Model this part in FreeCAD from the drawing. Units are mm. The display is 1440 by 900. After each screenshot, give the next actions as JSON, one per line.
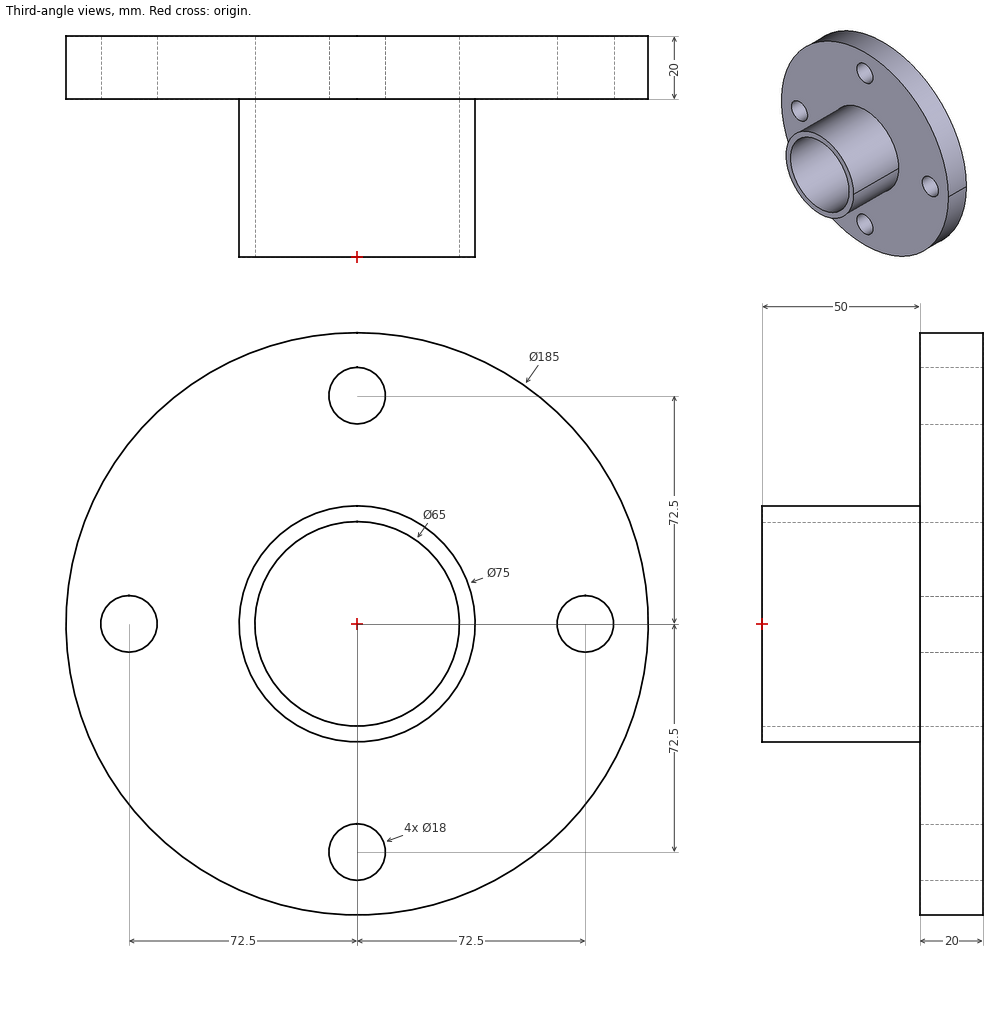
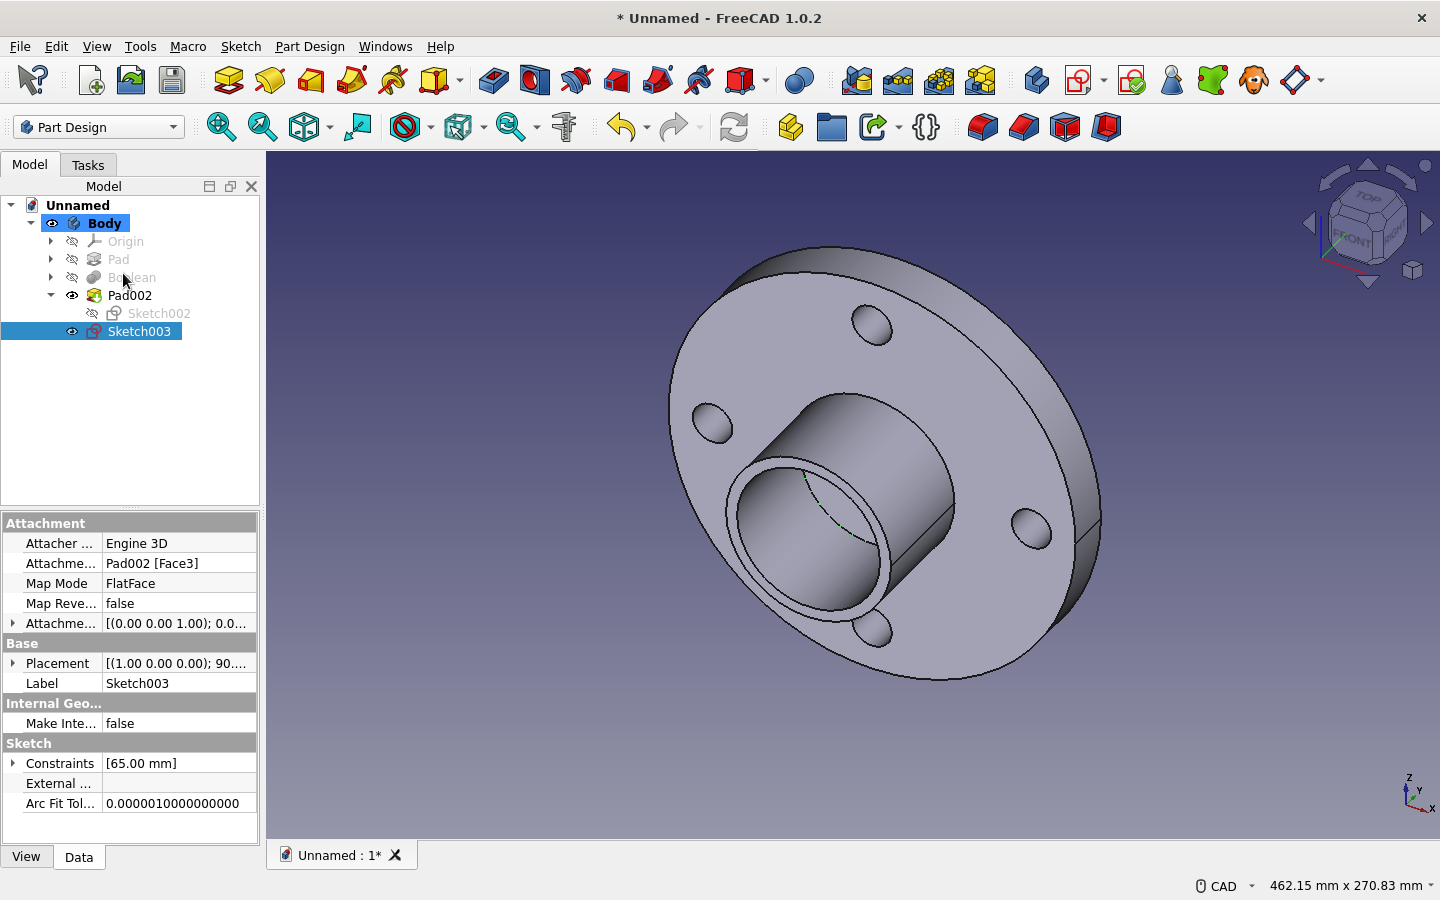
{"action": "left_click", "coordinate": [494, 80]}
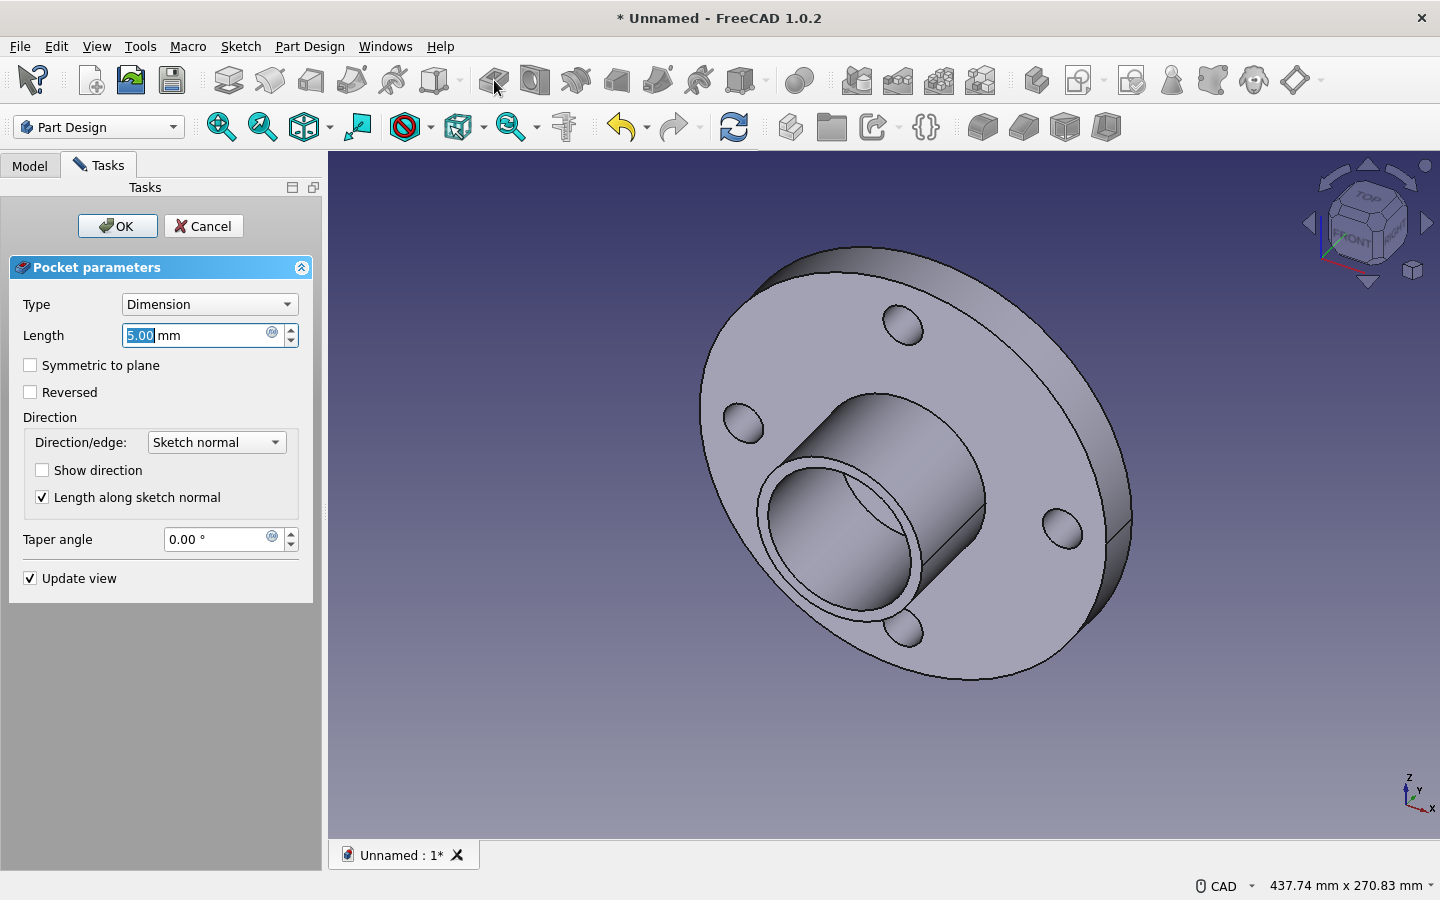
{"action": "left_click", "coordinate": [210, 304]}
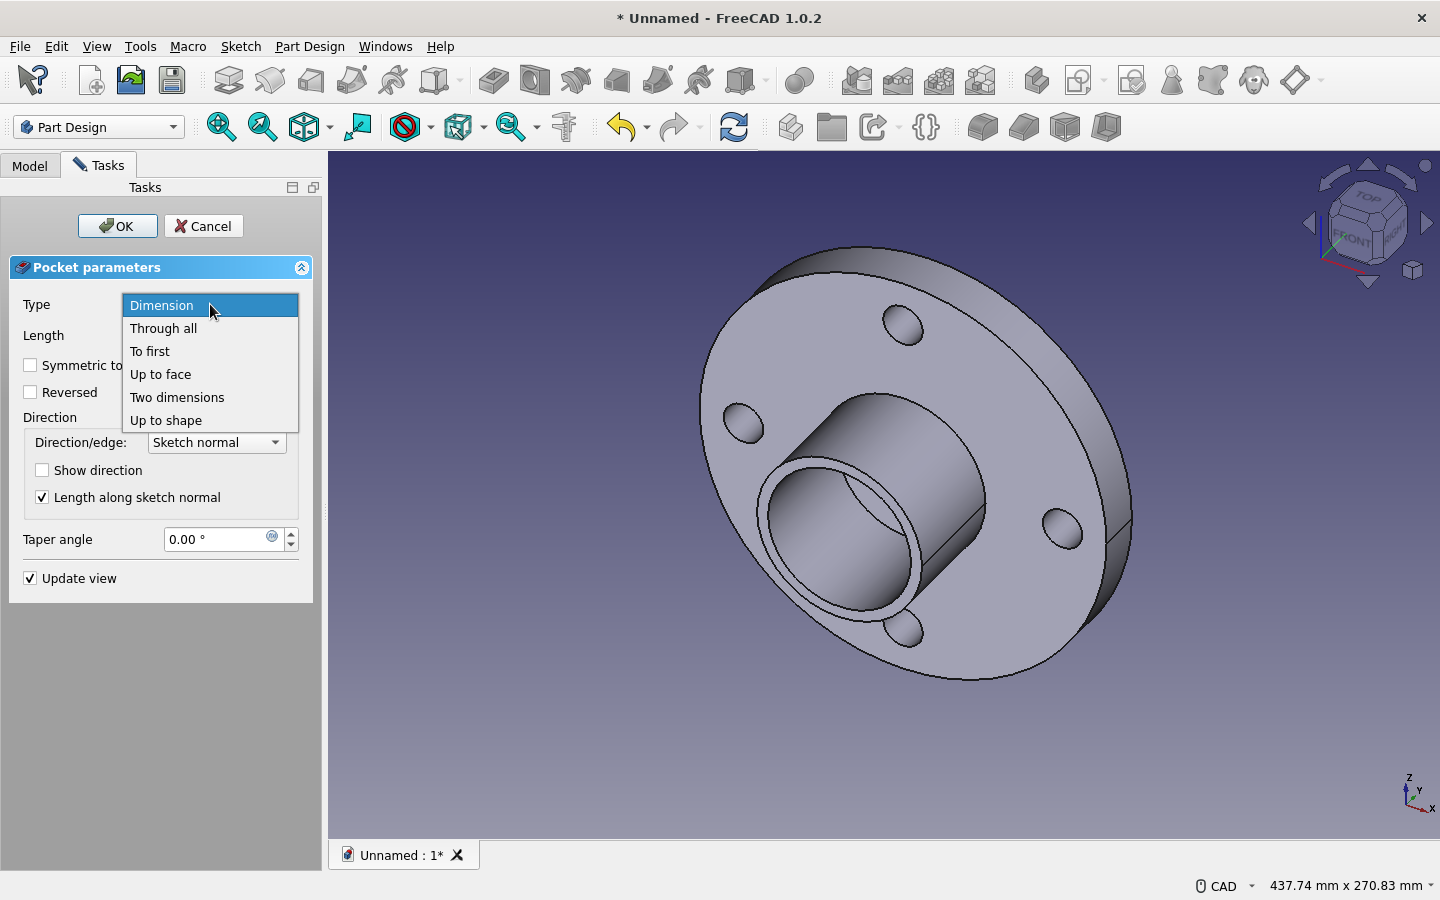
{"action": "left_click", "coordinate": [208, 328]}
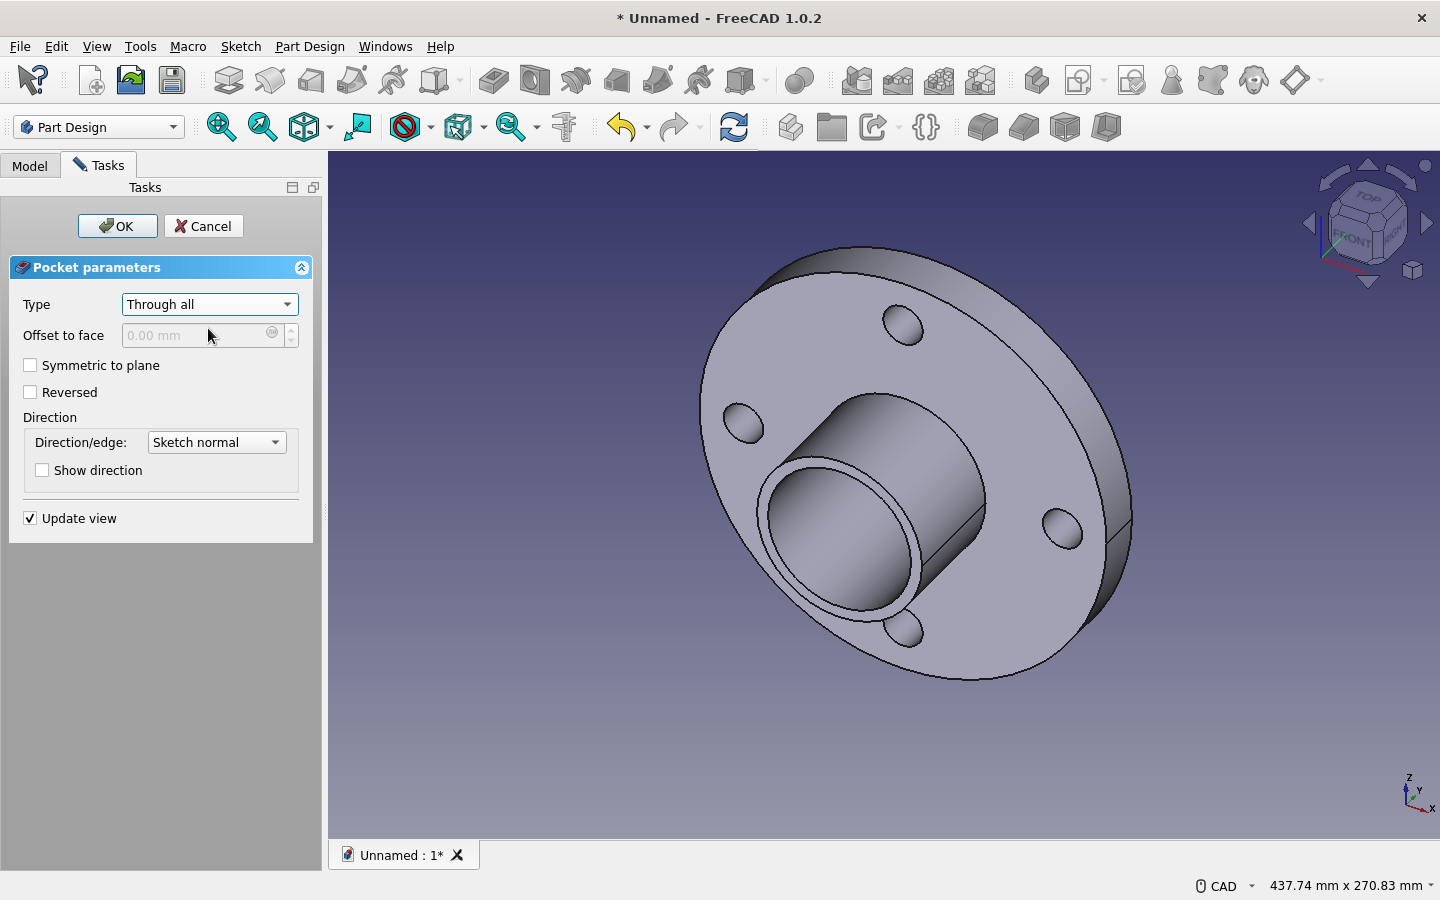
{"action": "left_click", "coordinate": [118, 226]}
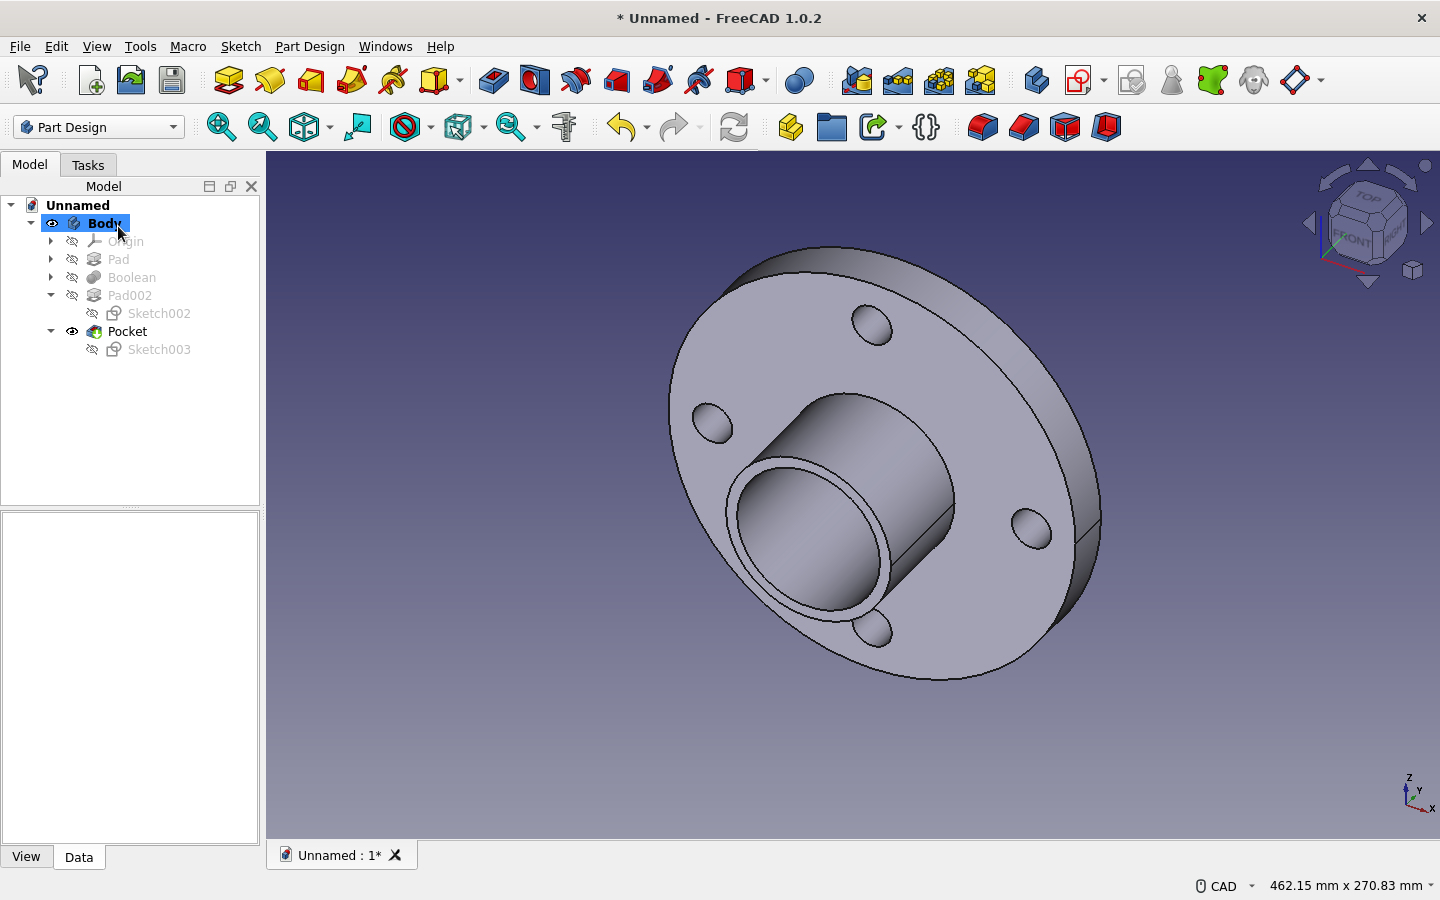
{"action": "key", "text": "0"}